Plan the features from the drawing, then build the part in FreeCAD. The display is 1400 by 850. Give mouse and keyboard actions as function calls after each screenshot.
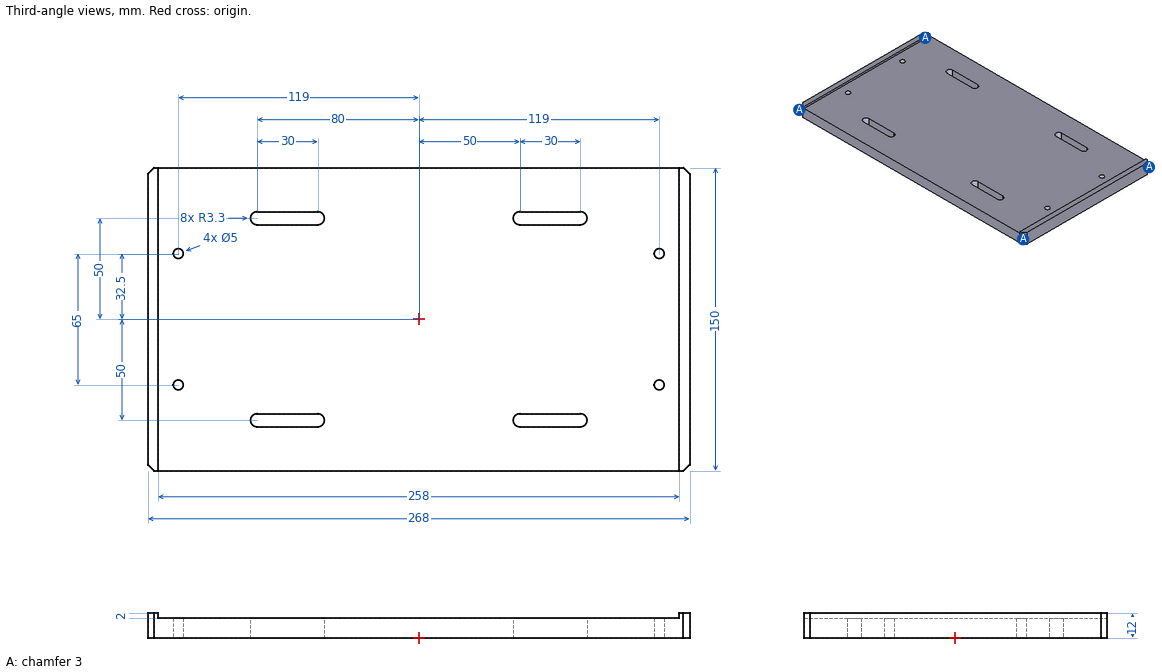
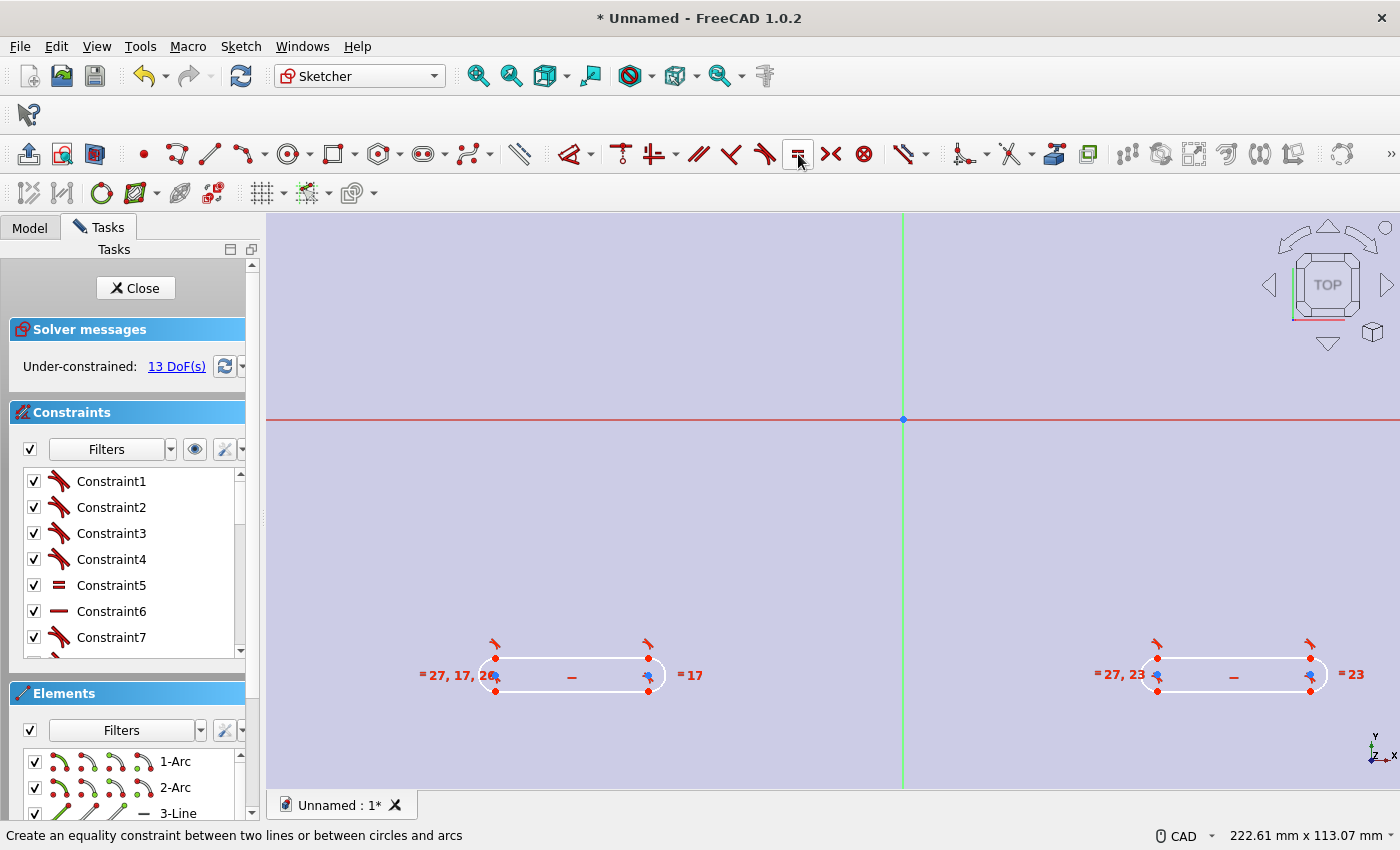
scroll(482, 667, down, 2)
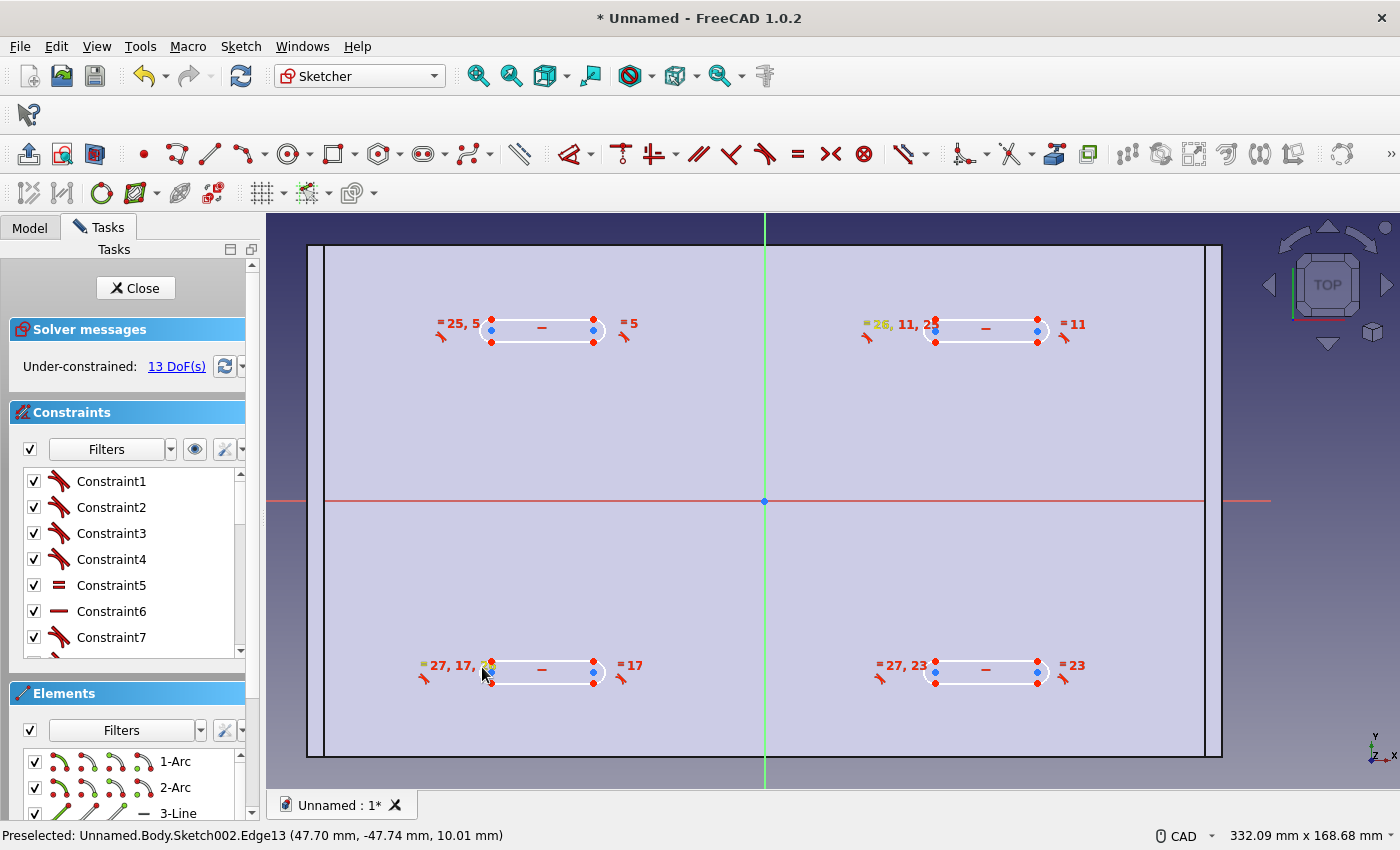
scroll(482, 324, up, 7)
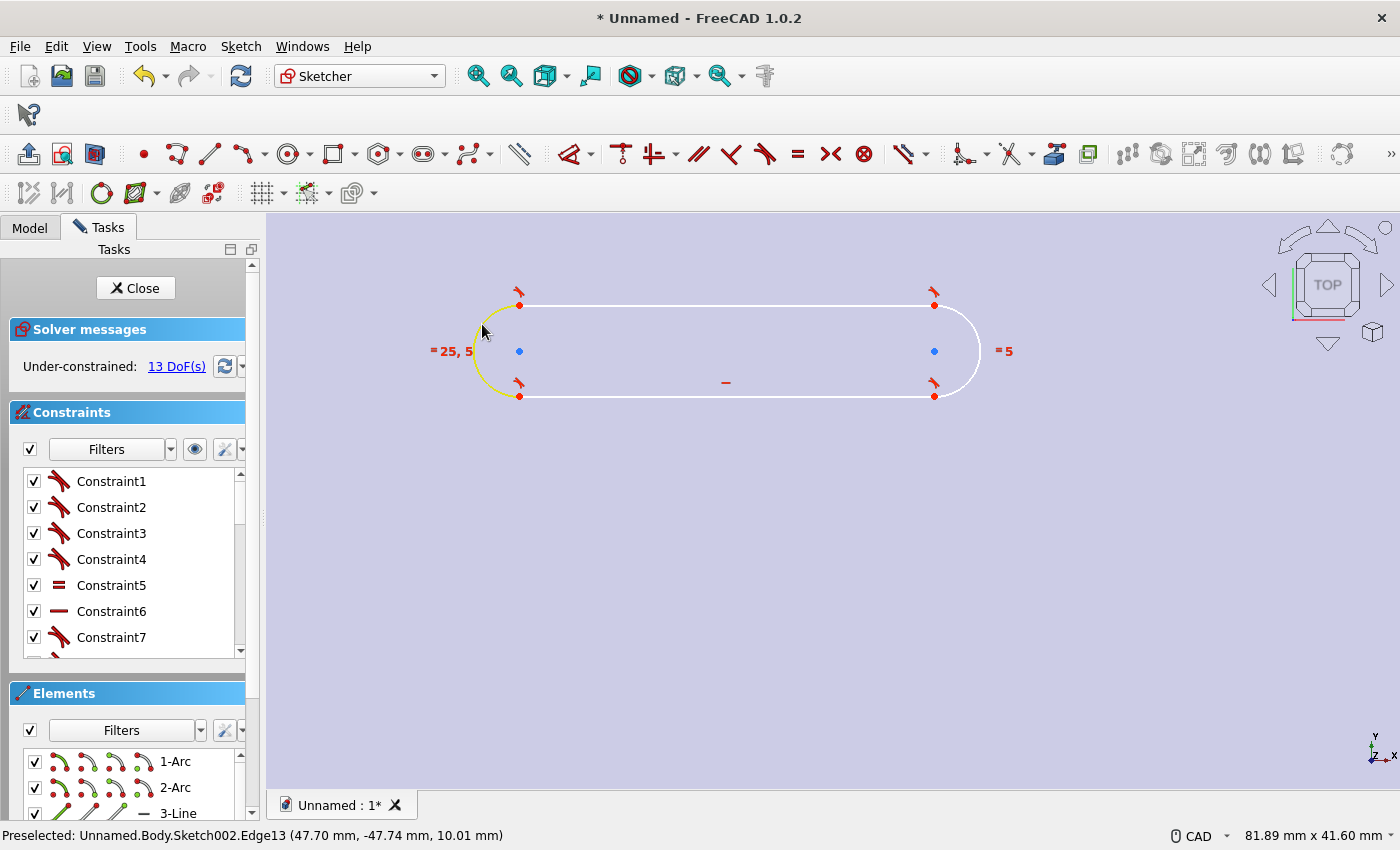
click(482, 325)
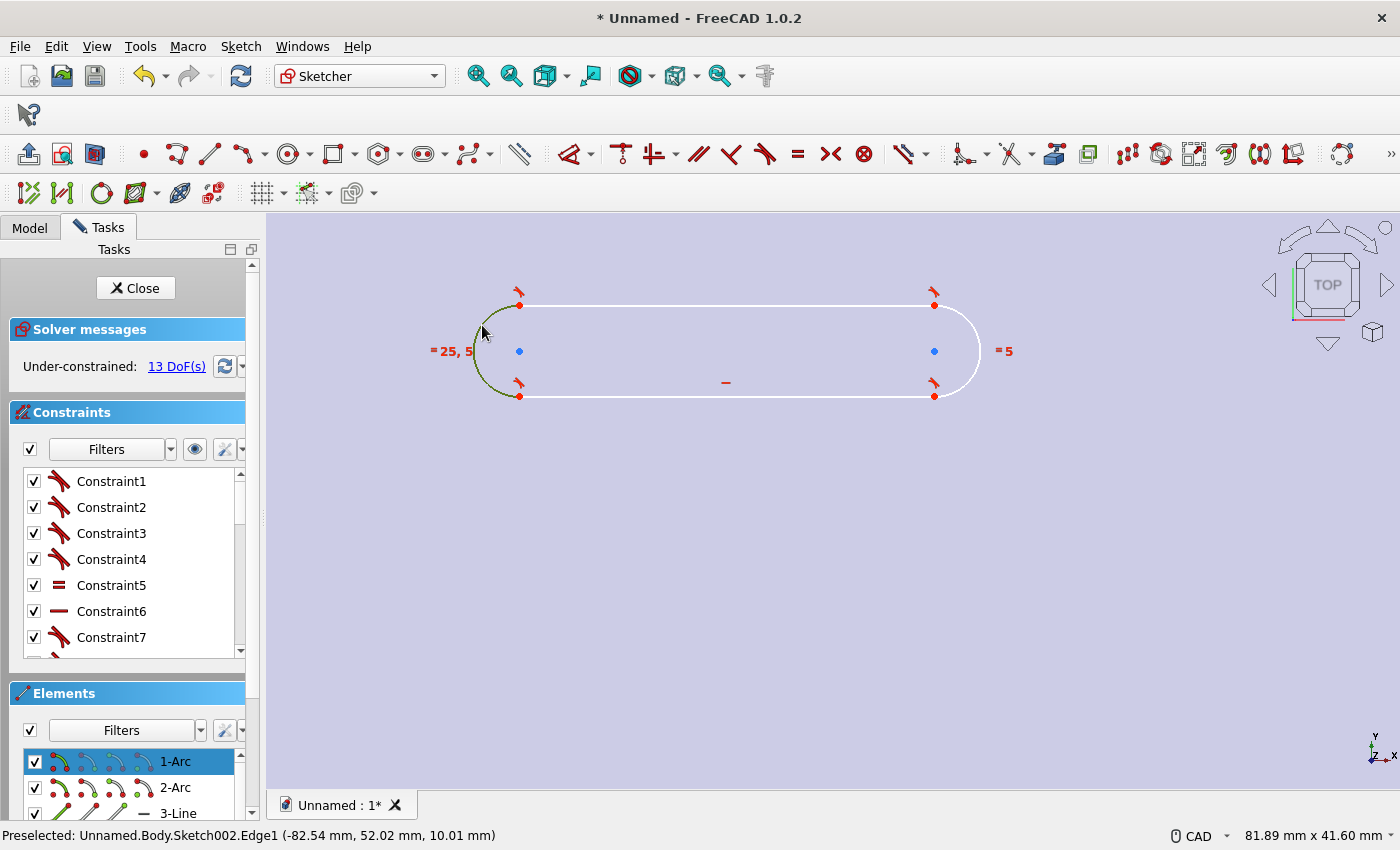
key(k)
key(r)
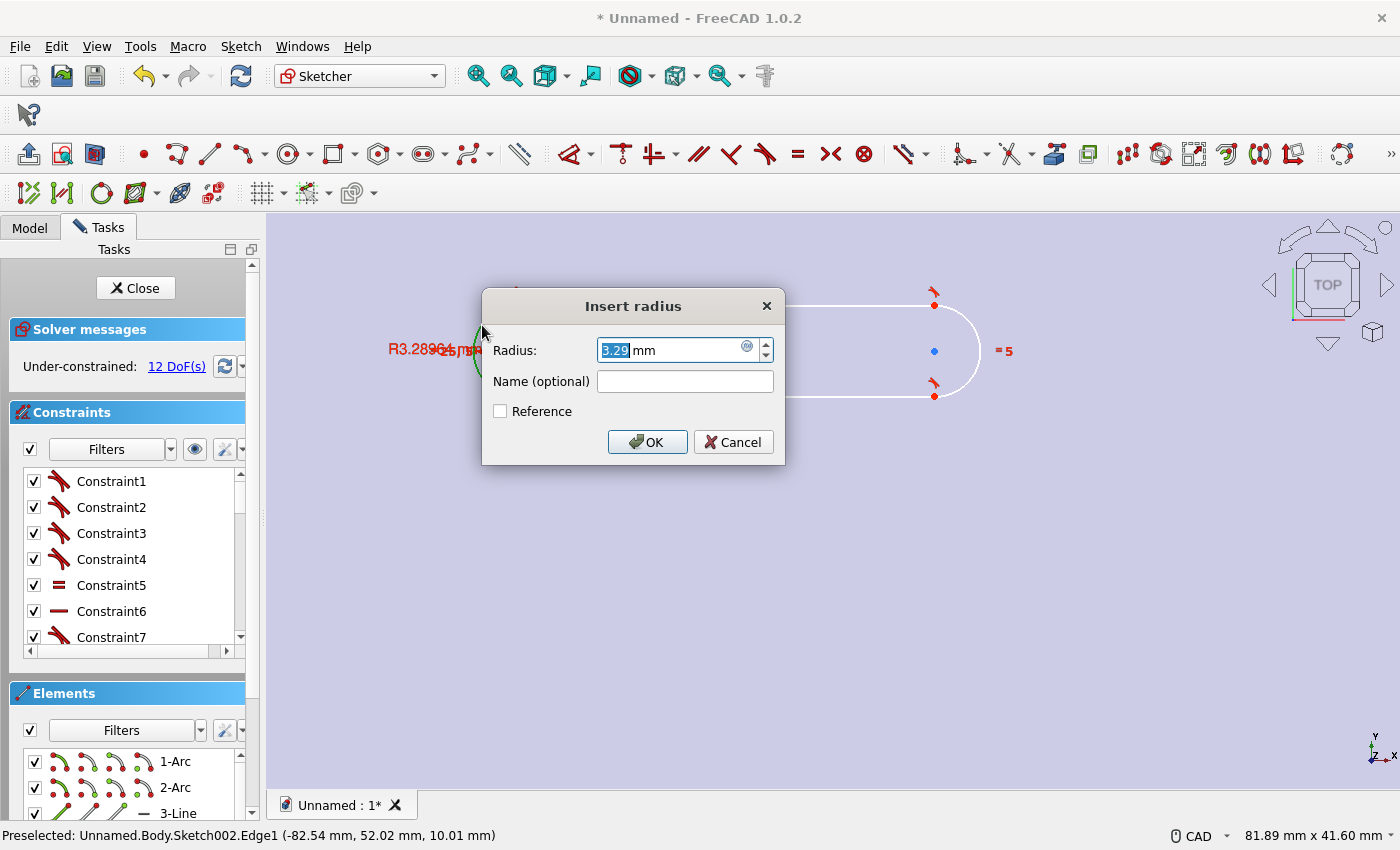
text(3.3)
key(Return)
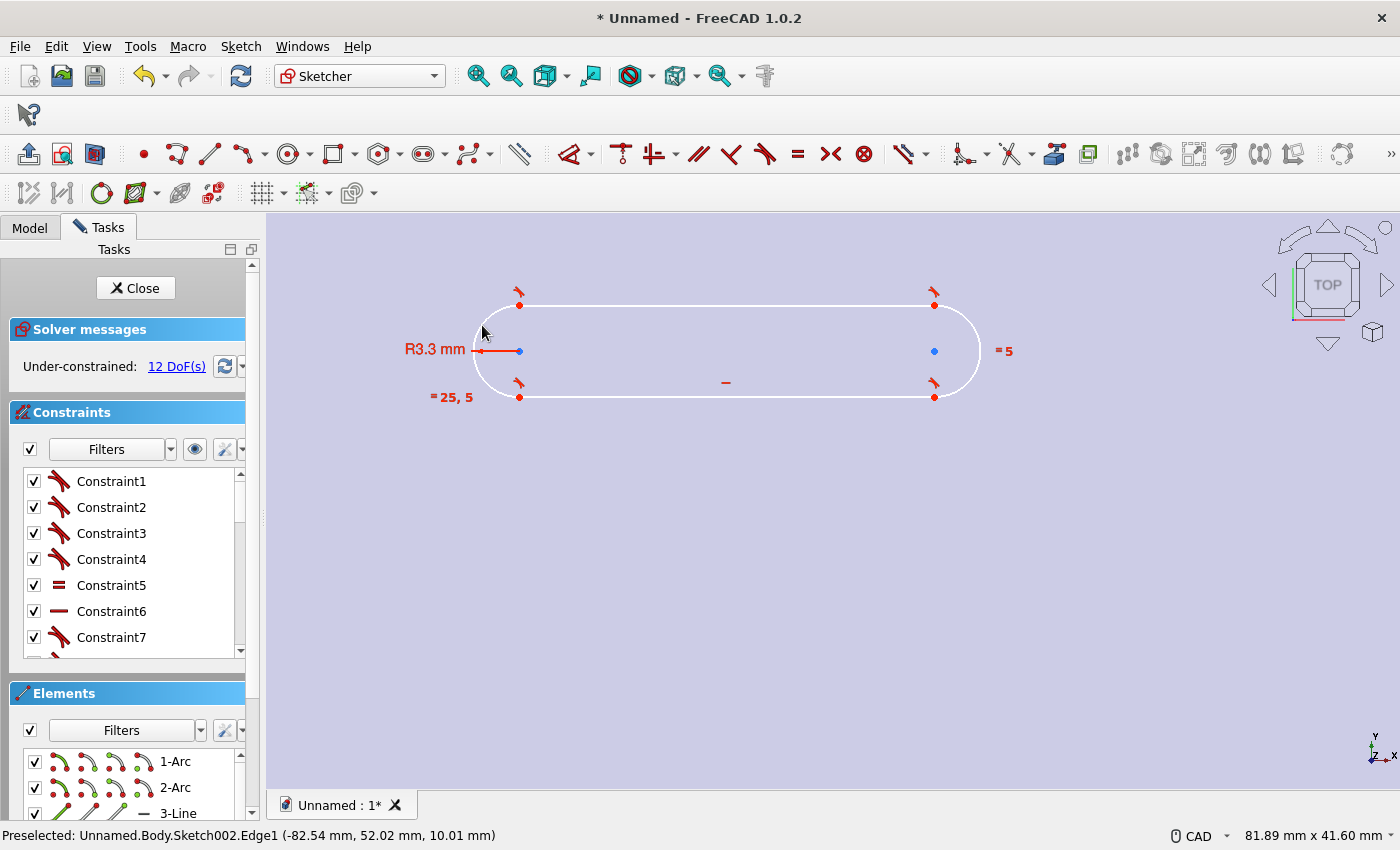
scroll(482, 324, down, 7)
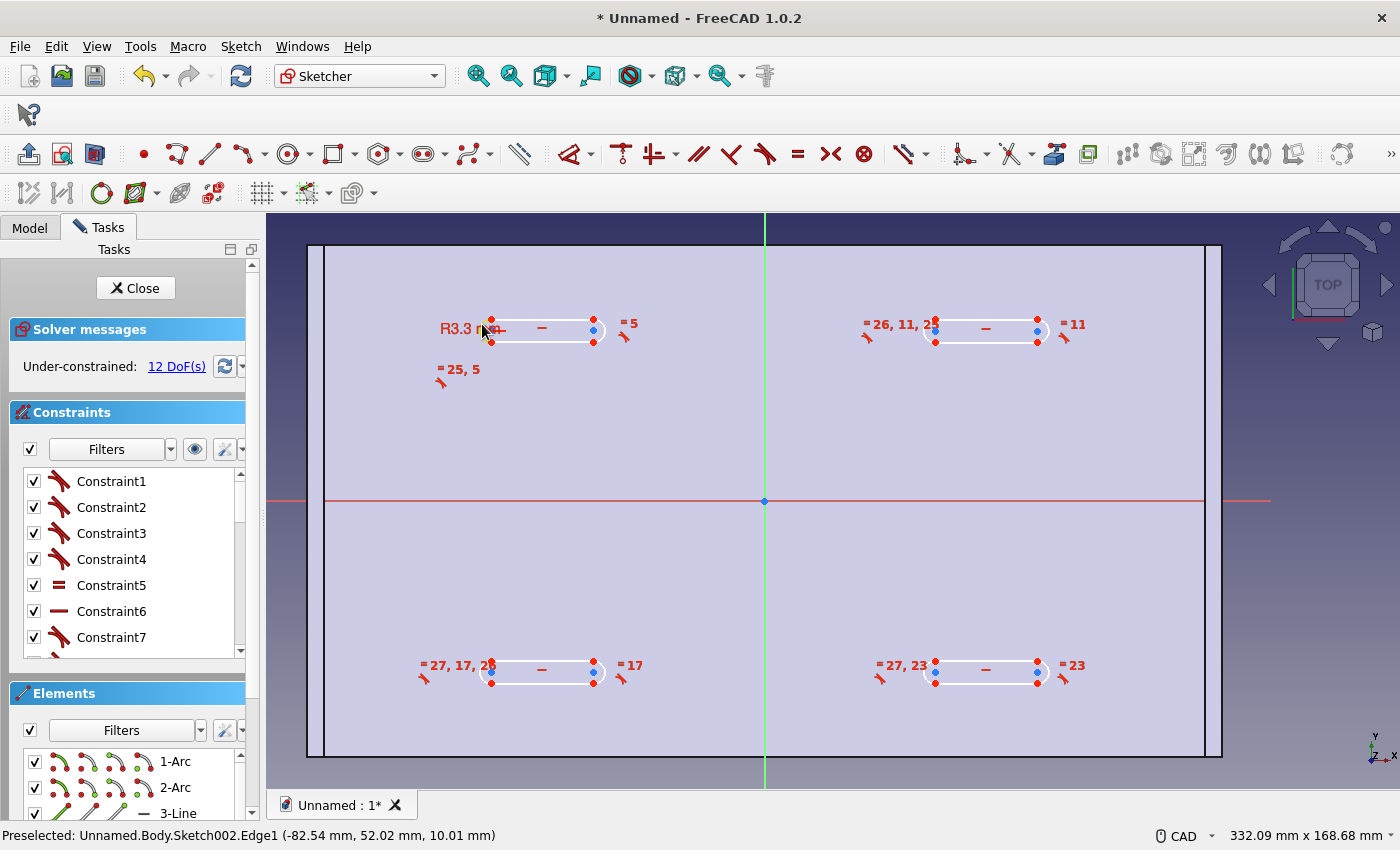
click(522, 320)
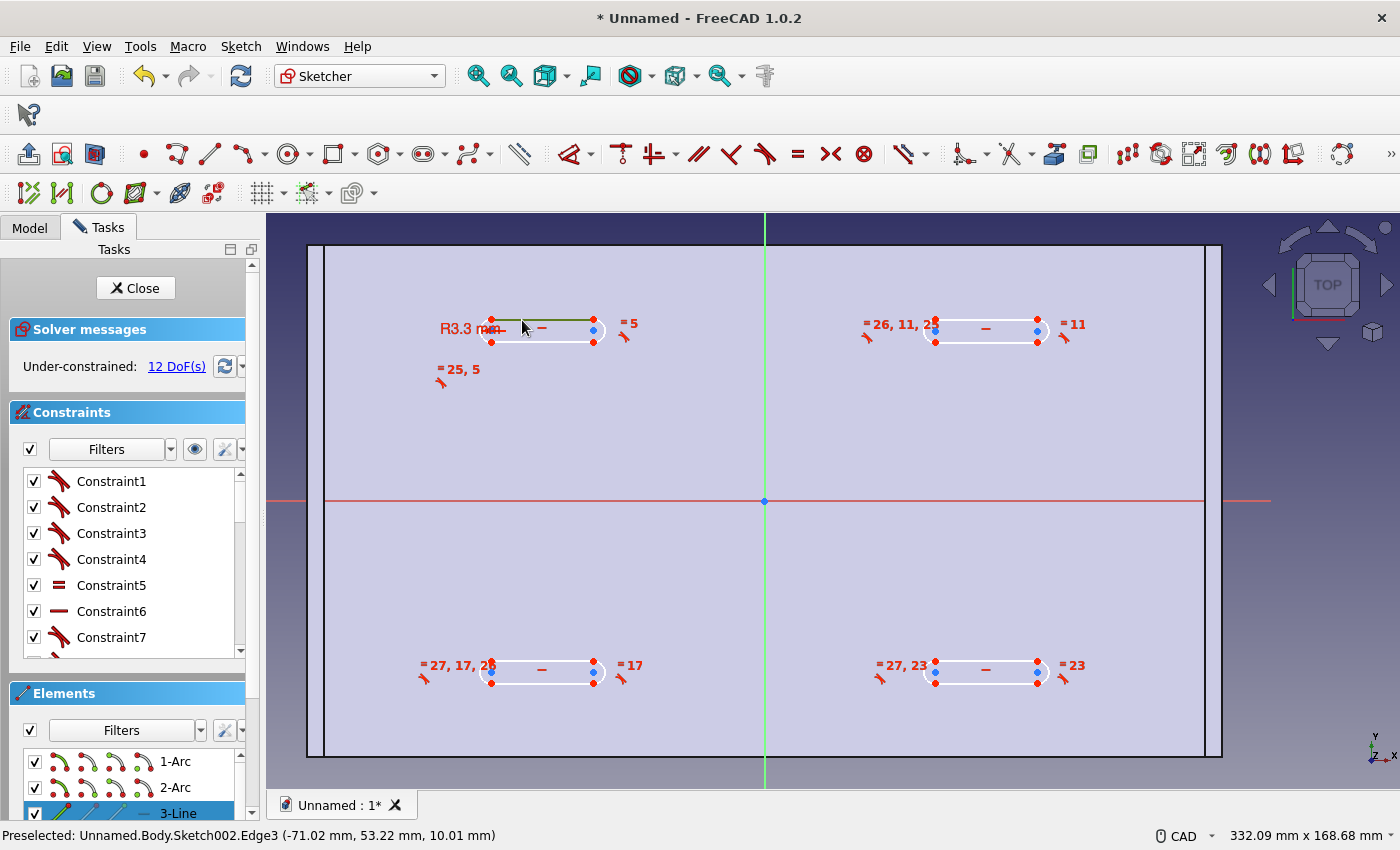
click(590, 154)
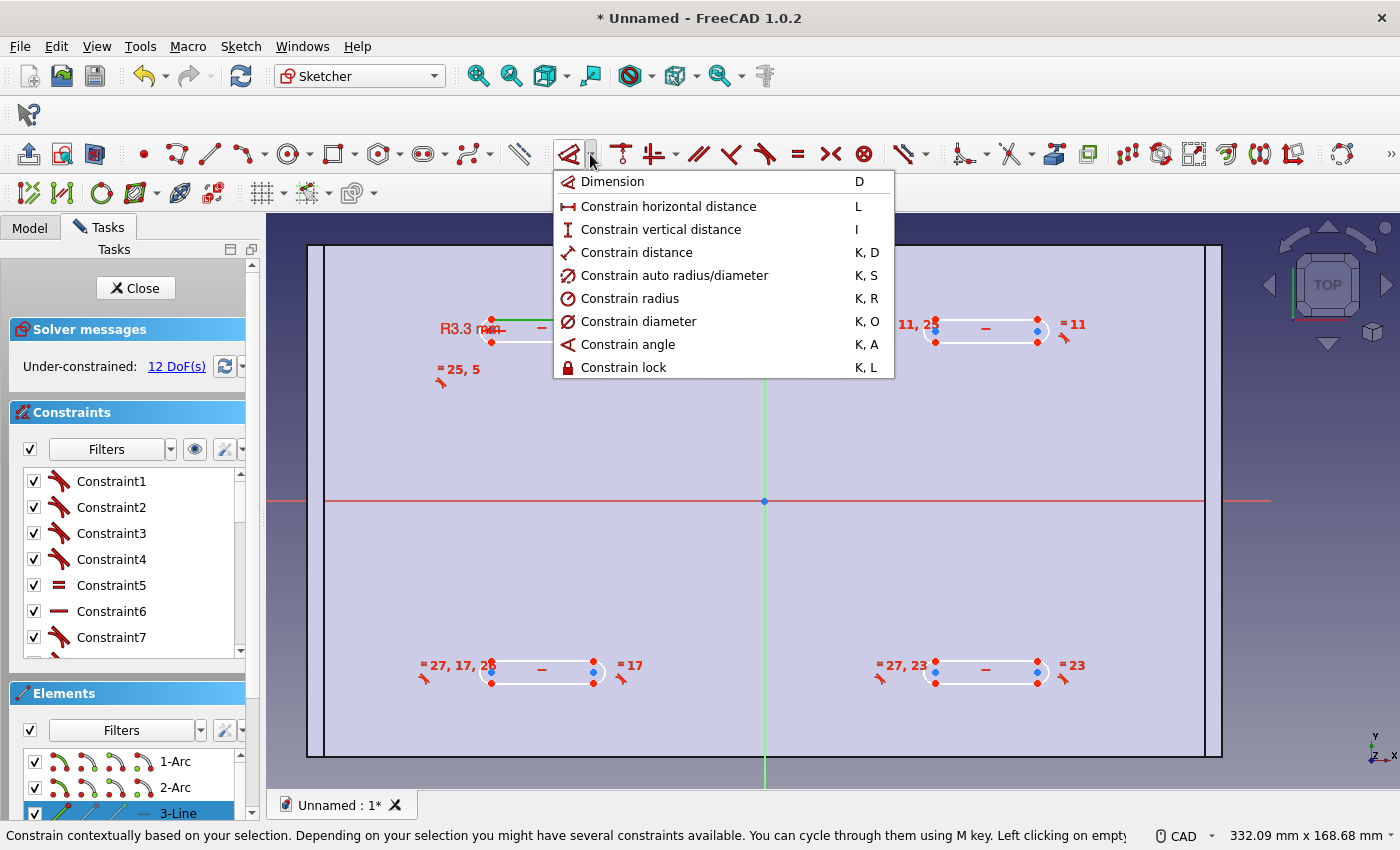
click(724, 206)